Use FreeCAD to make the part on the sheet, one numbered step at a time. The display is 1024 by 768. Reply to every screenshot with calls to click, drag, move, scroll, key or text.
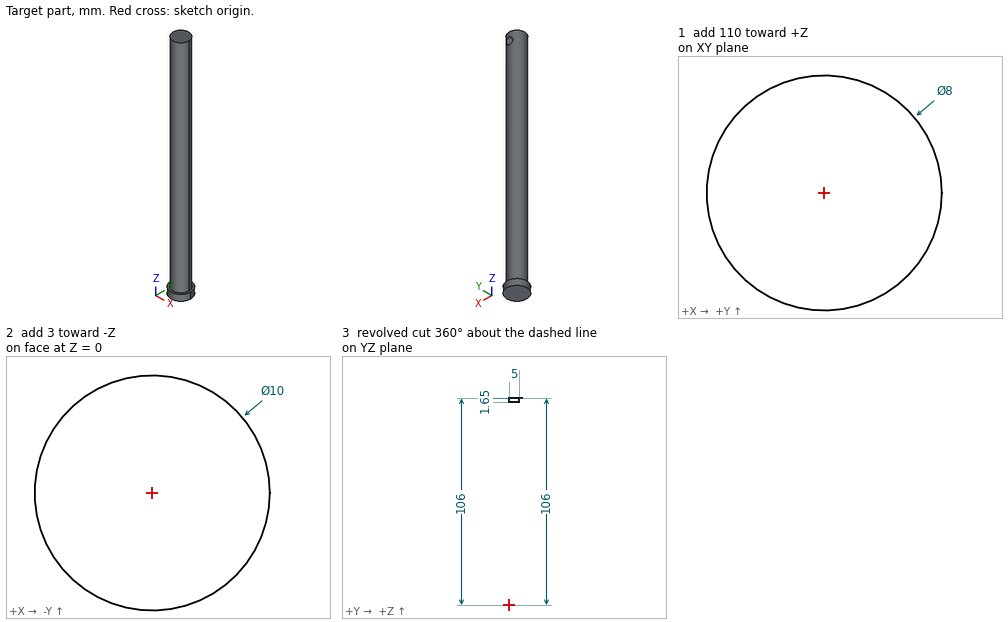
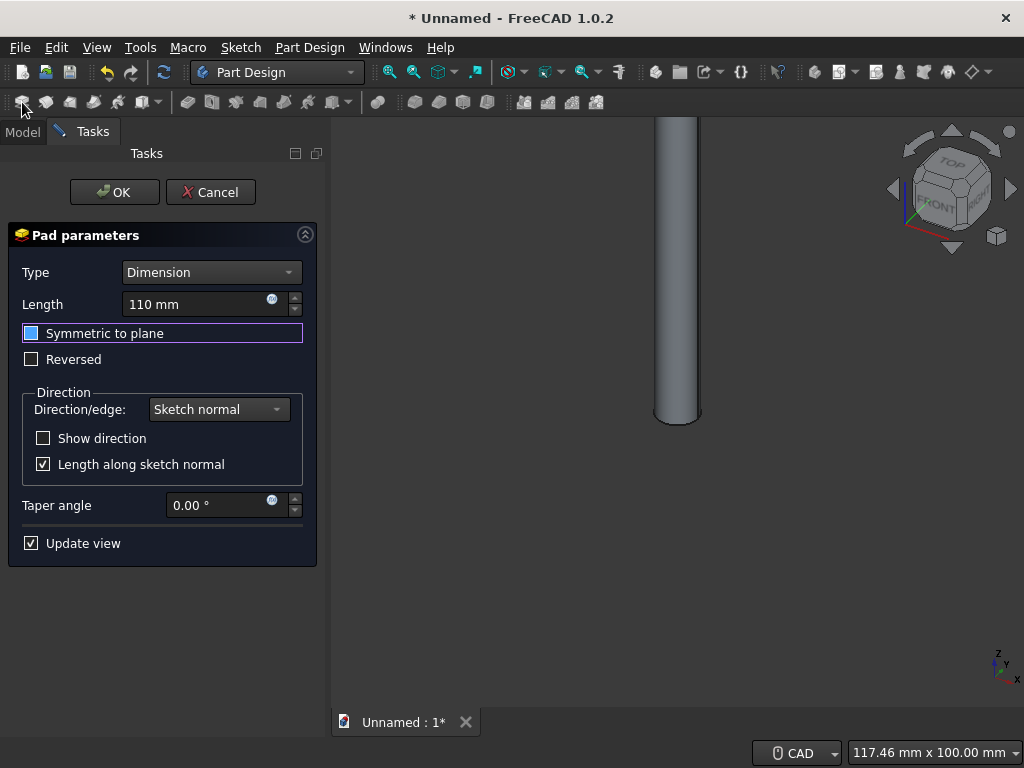
click(115, 192)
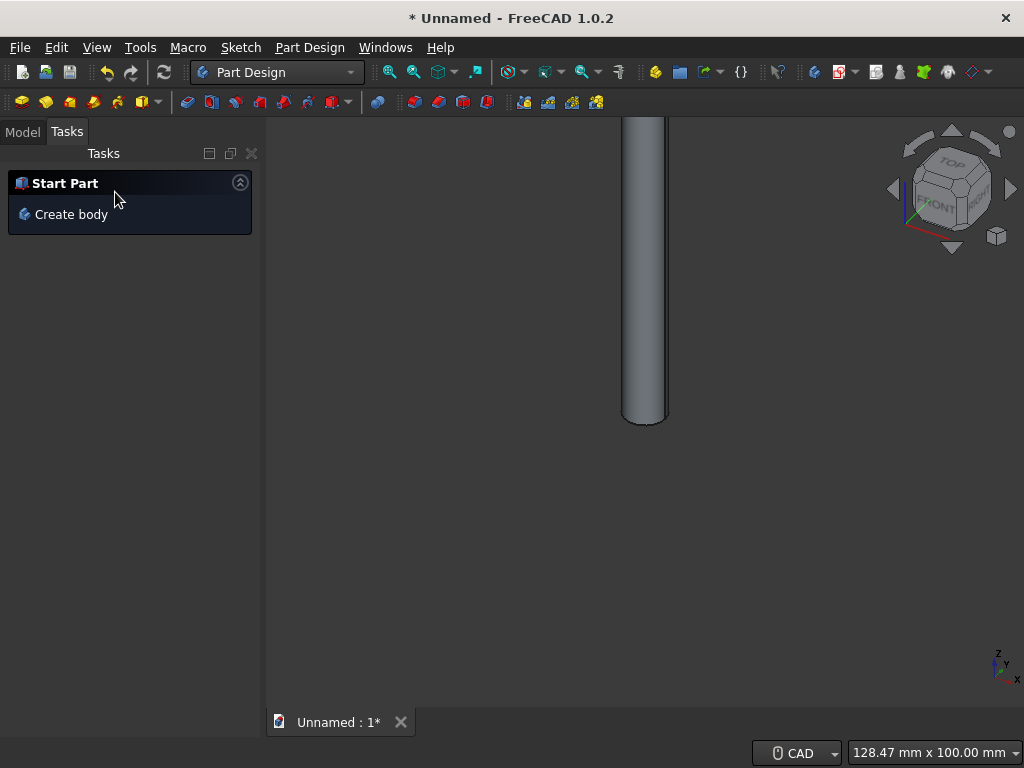
click(390, 72)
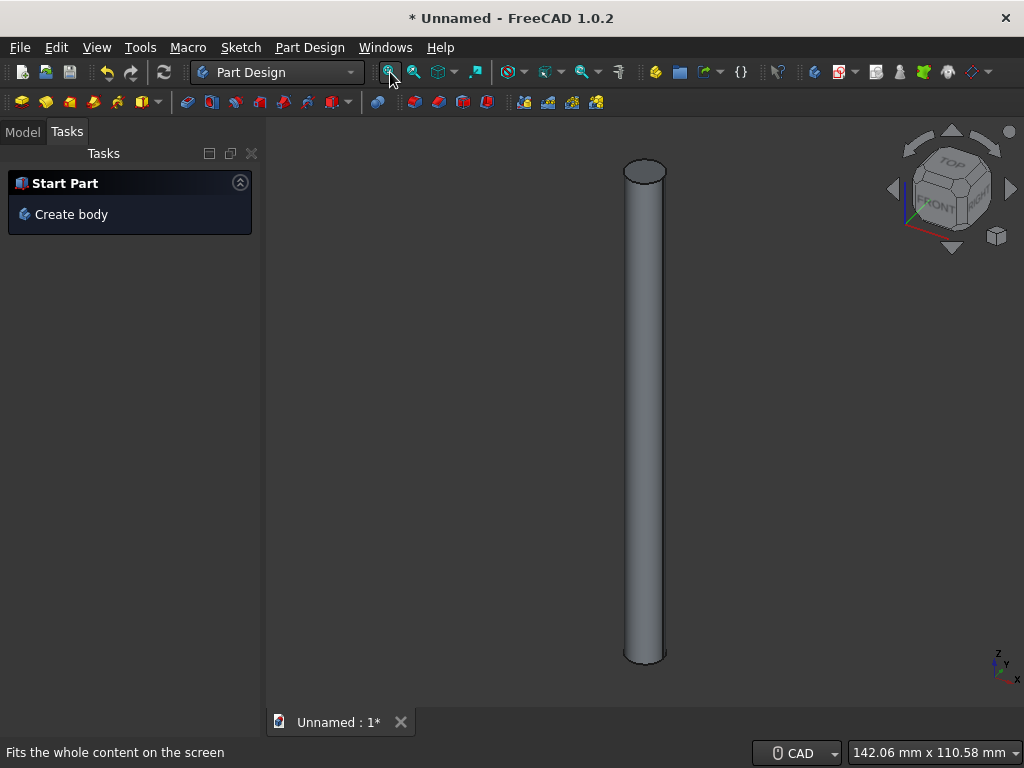
key(5)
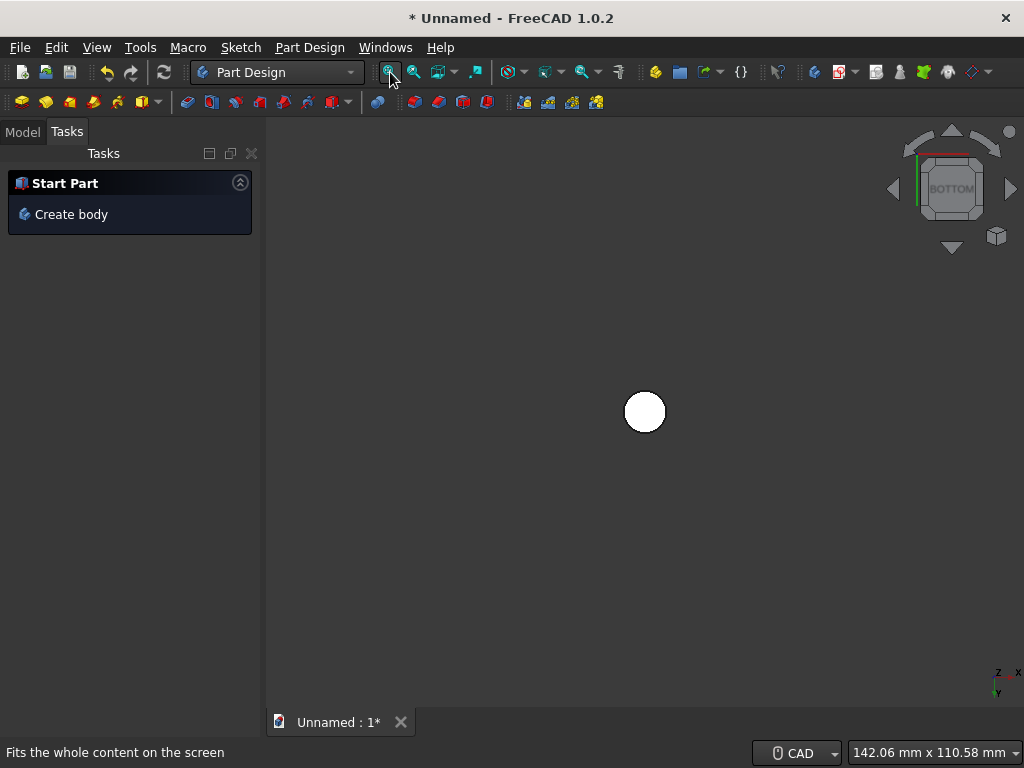
click(390, 72)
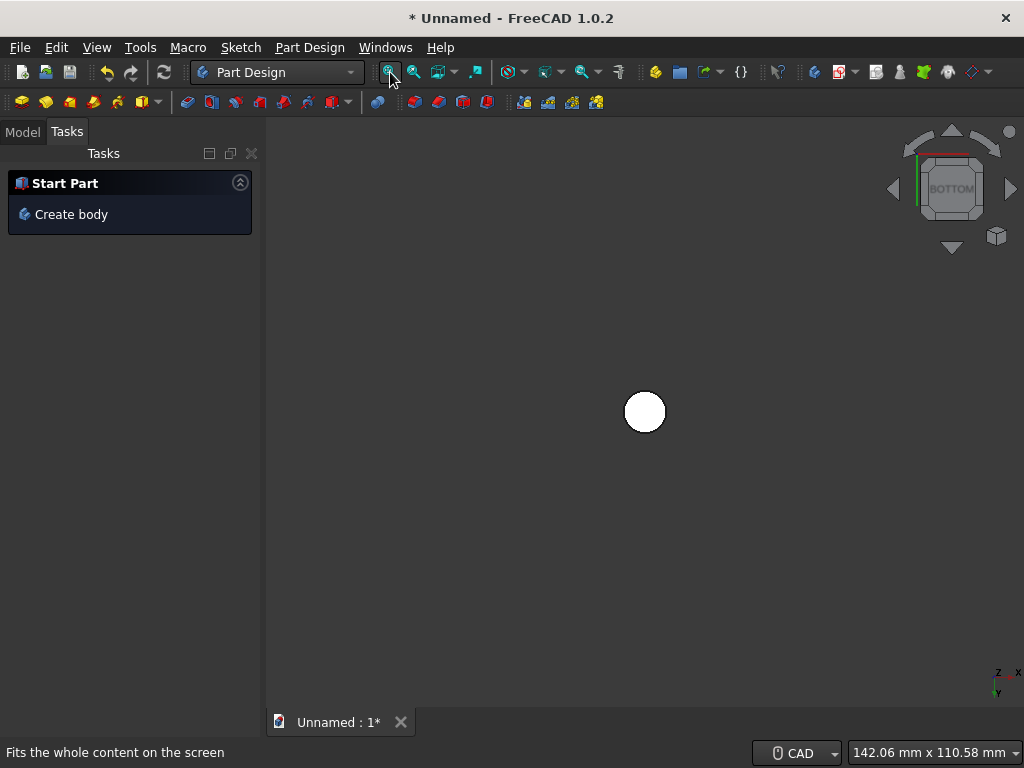
click(645, 411)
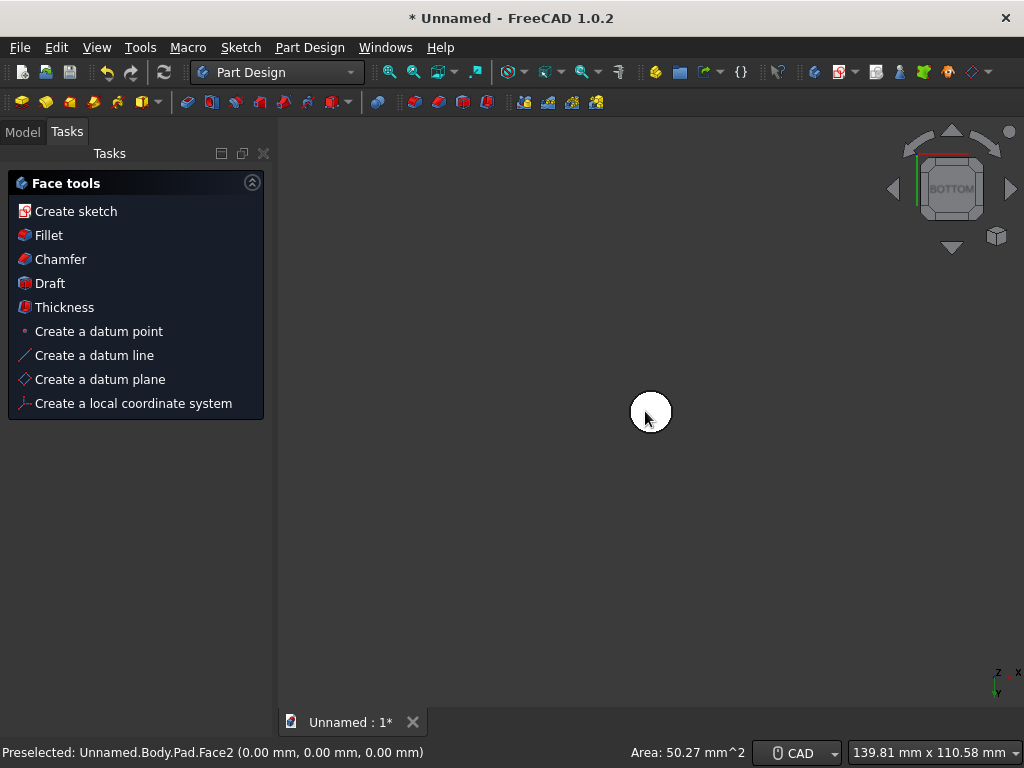
click(840, 72)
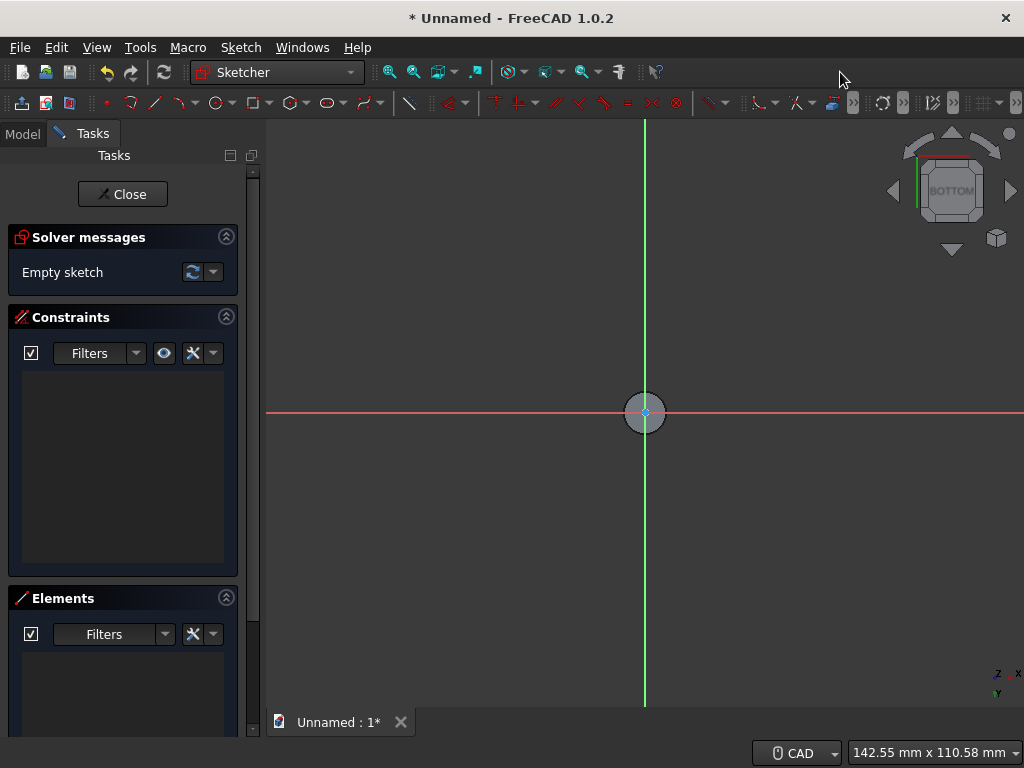
scroll(656, 413, up, 10)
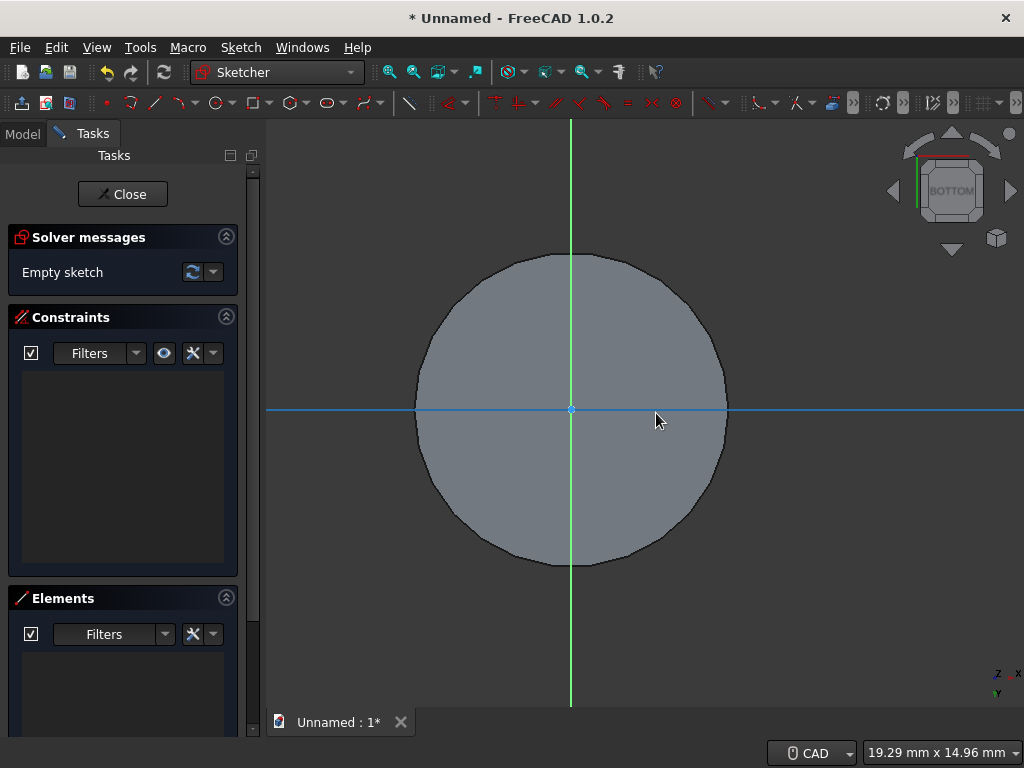
click(216, 104)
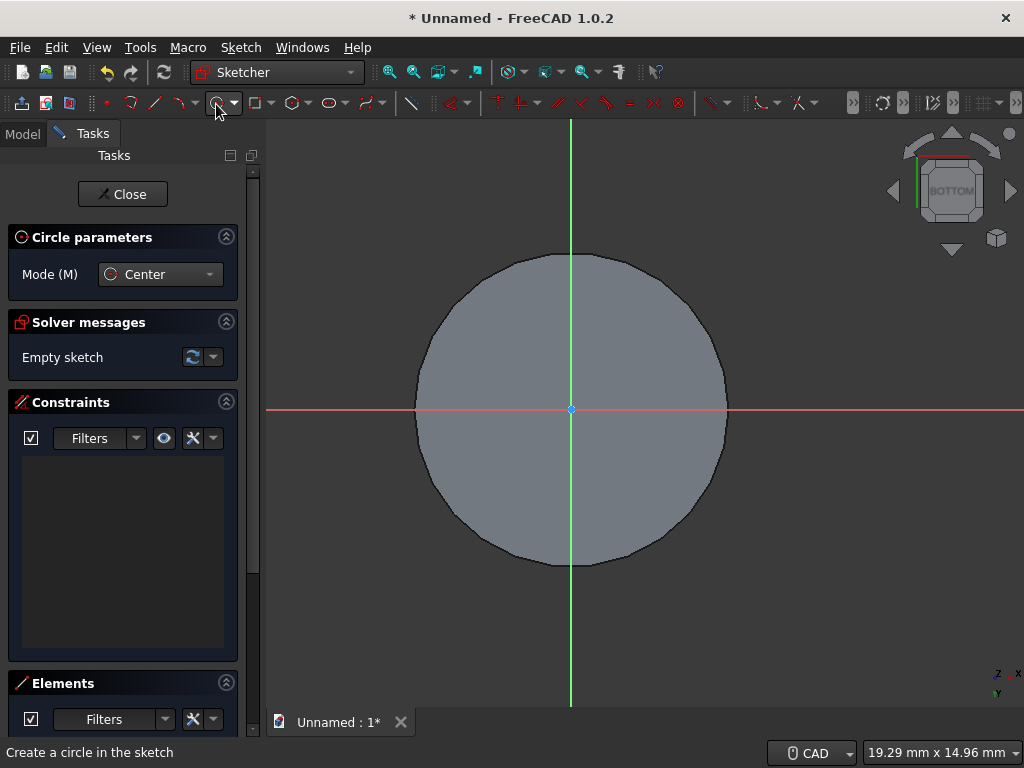
click(571, 410)
click(710, 271)
key(Escape)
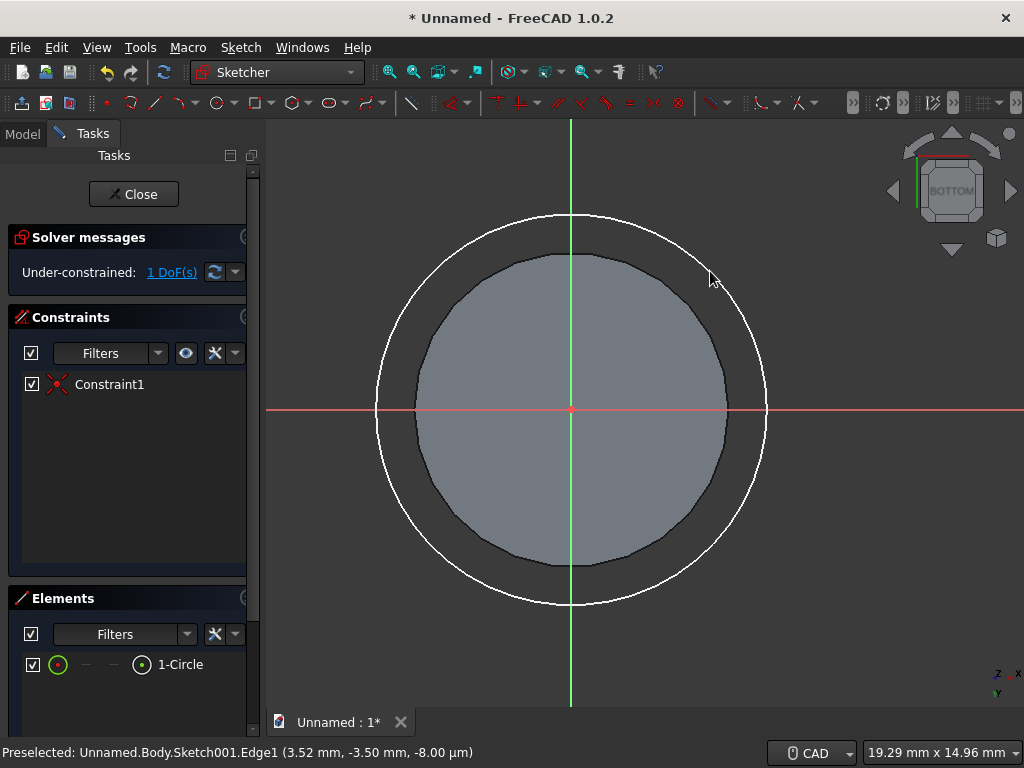
click(450, 104)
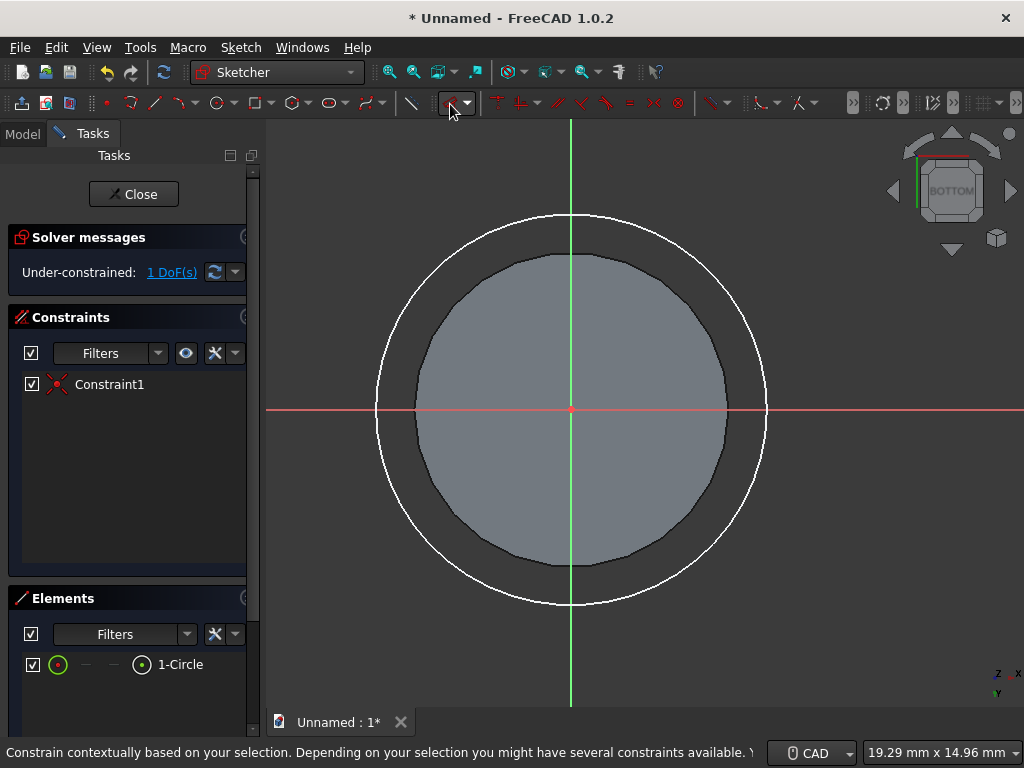
click(709, 271)
click(732, 248)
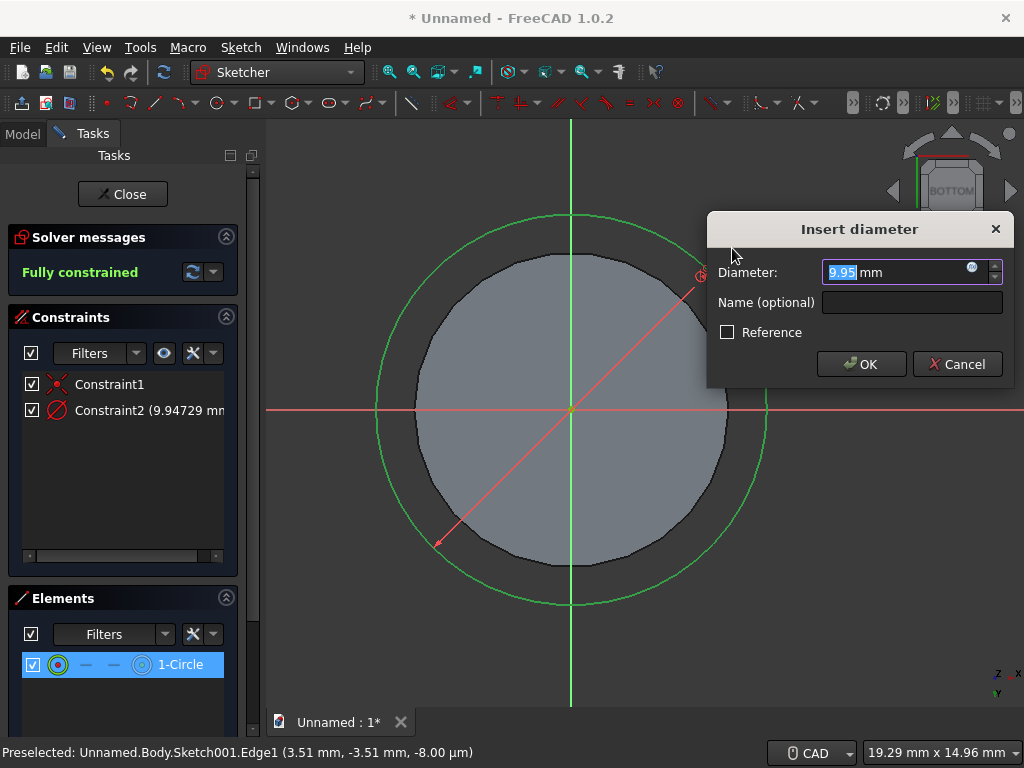
text(10)
key(Return)
key(Escape)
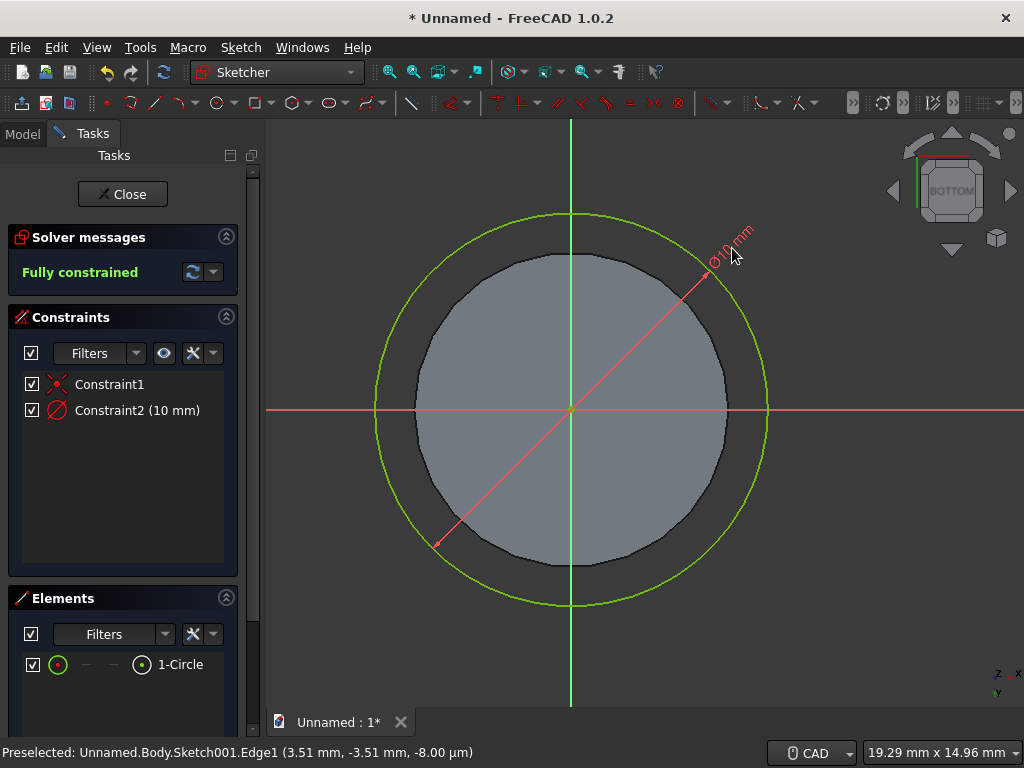
click(123, 194)